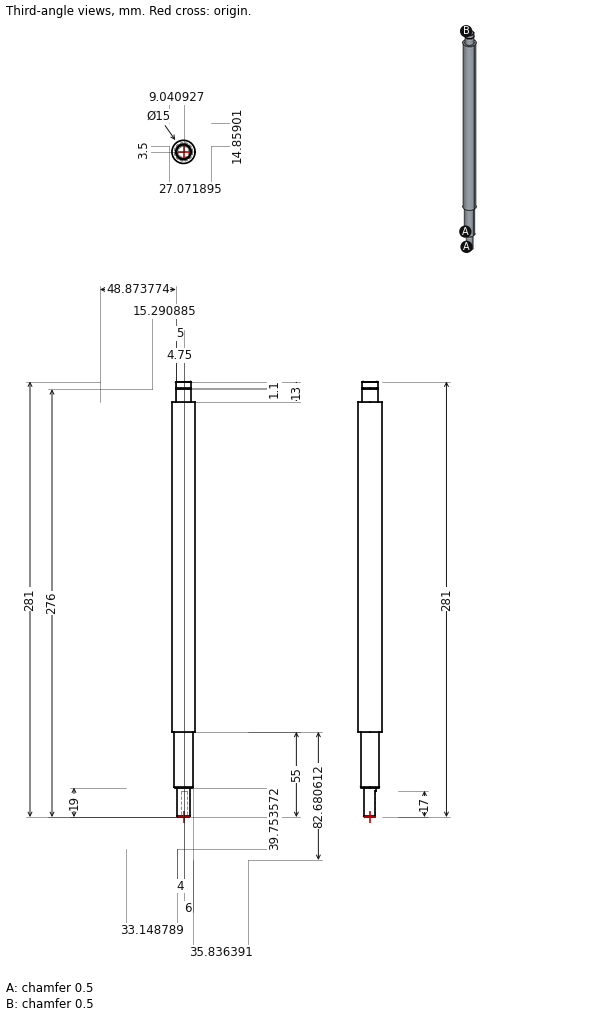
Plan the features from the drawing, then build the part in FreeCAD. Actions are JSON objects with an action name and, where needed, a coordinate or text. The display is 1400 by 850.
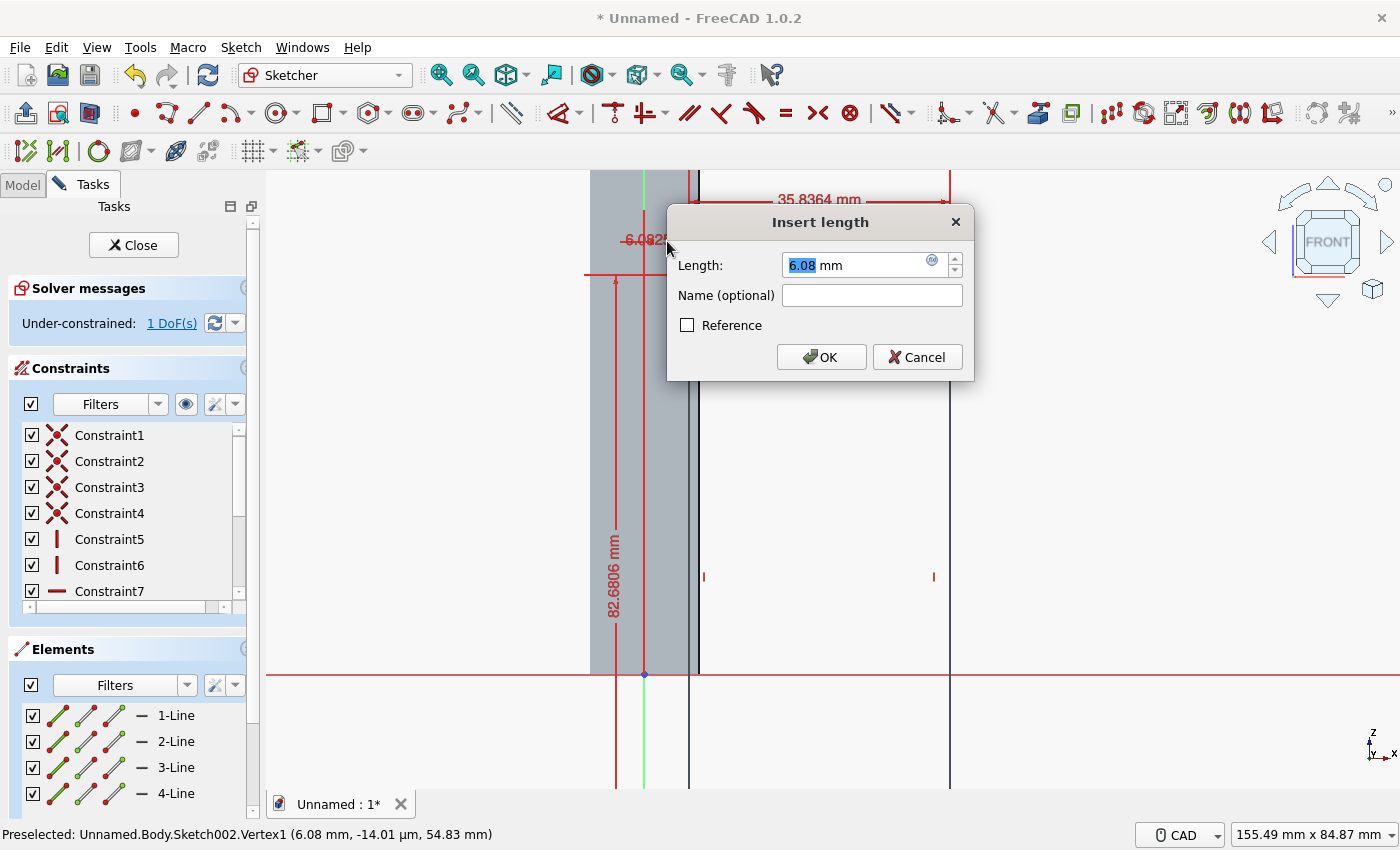
{"action": "type", "text": "6"}
{"action": "key", "text": "Return"}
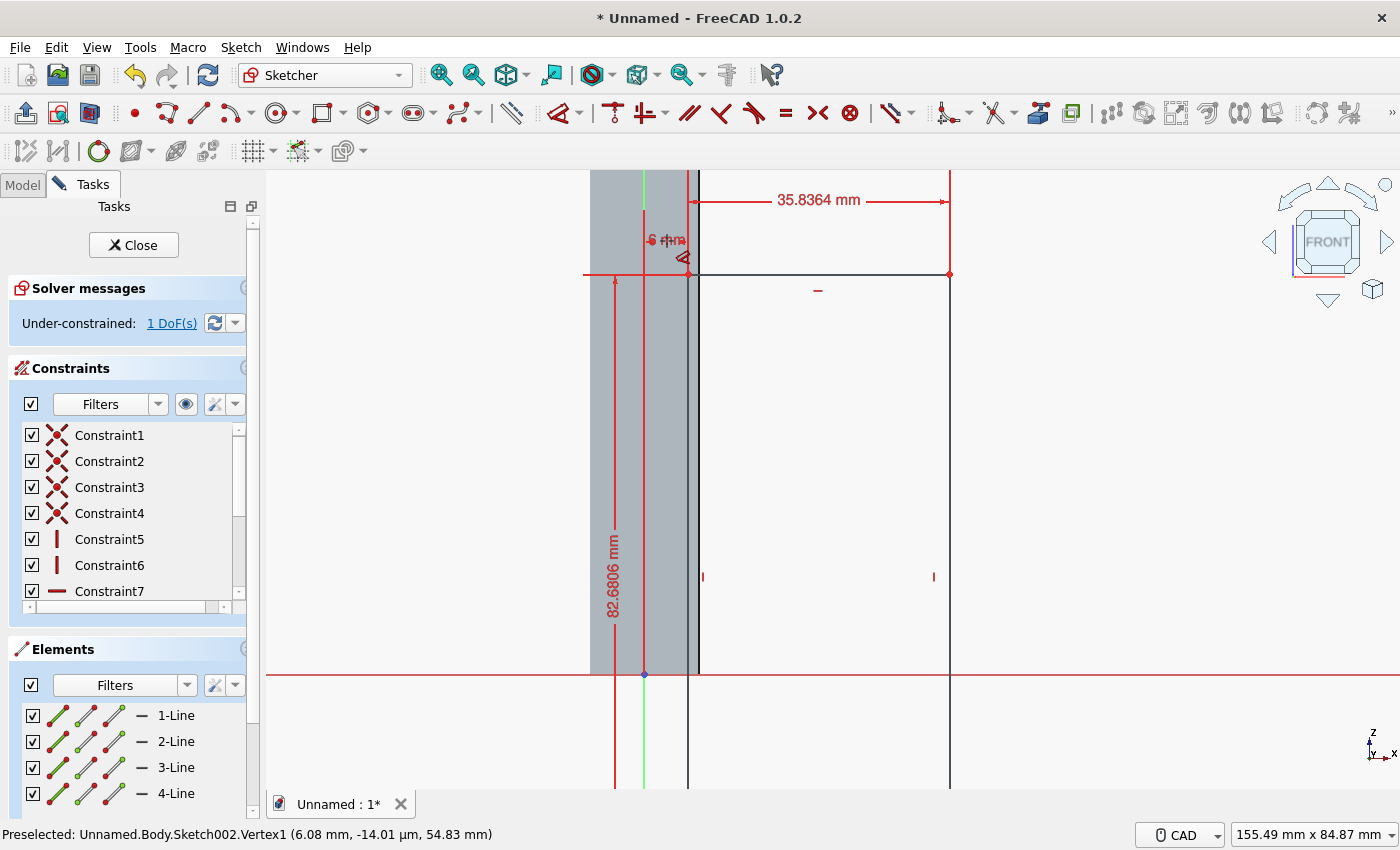
{"action": "left_click", "coordinate": [688, 275]}
{"action": "left_click", "coordinate": [610, 475]}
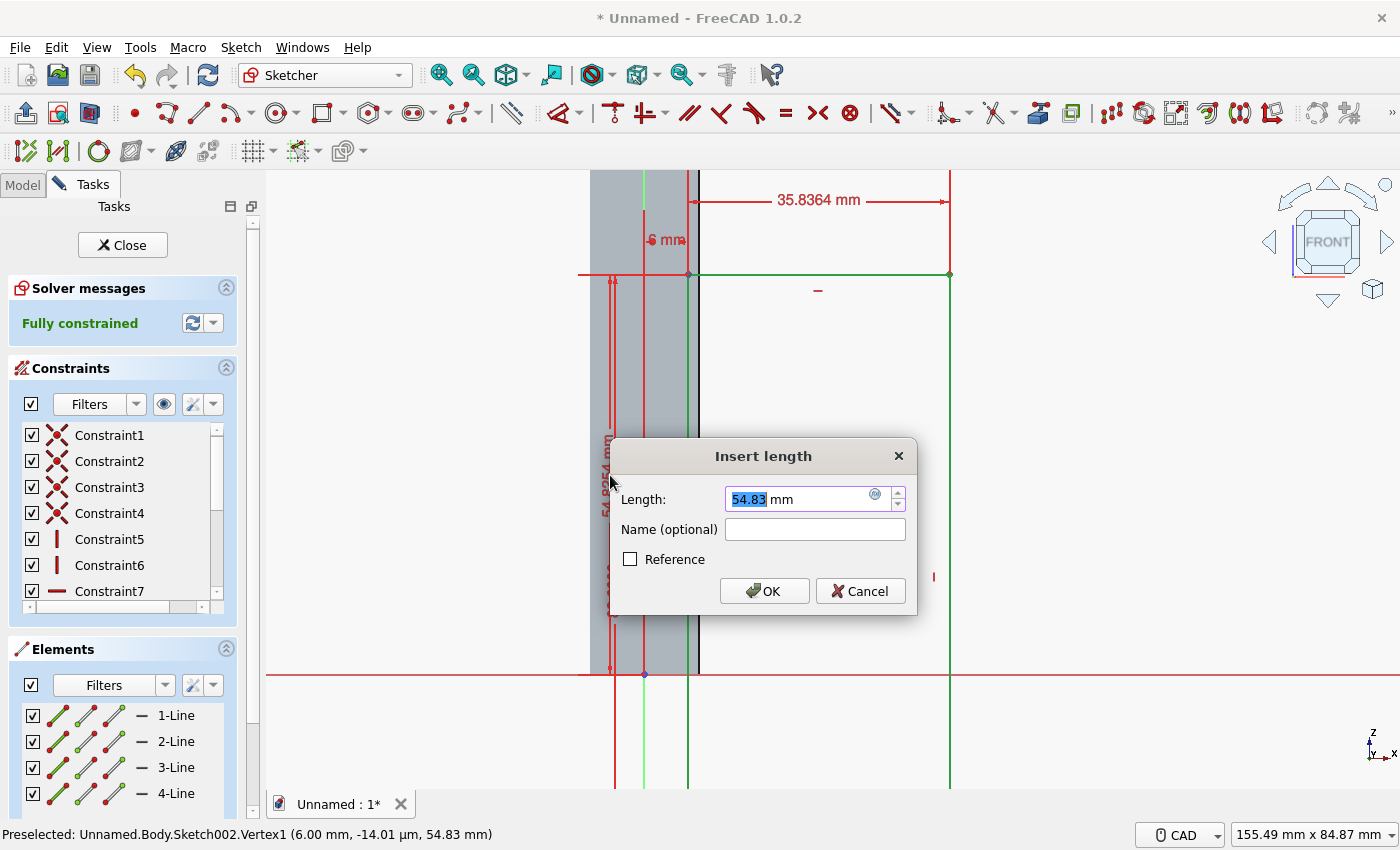
{"action": "type", "text": "55"}
{"action": "key", "text": "Return"}
{"action": "key", "text": "Escape"}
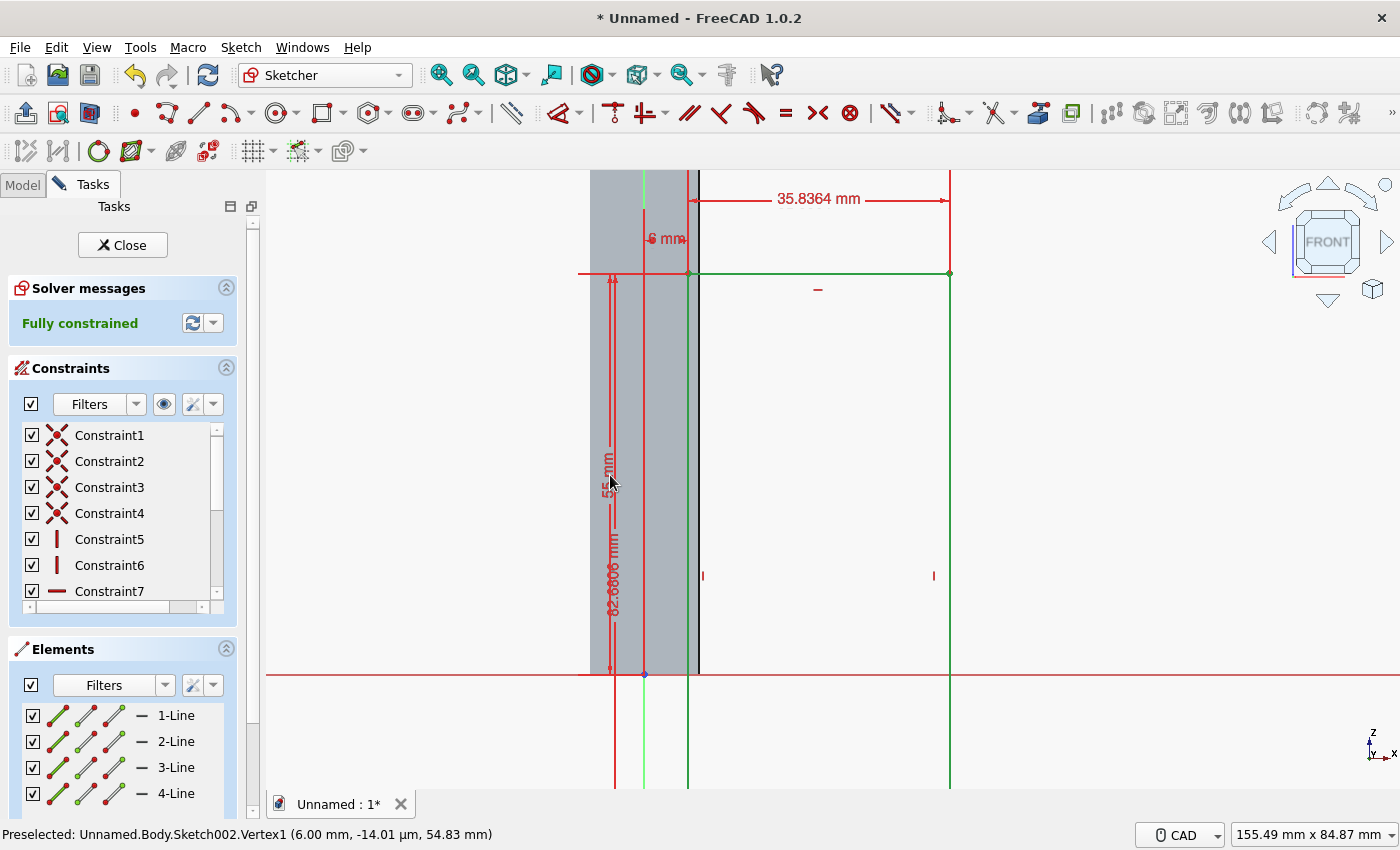
{"action": "left_click", "coordinate": [123, 245]}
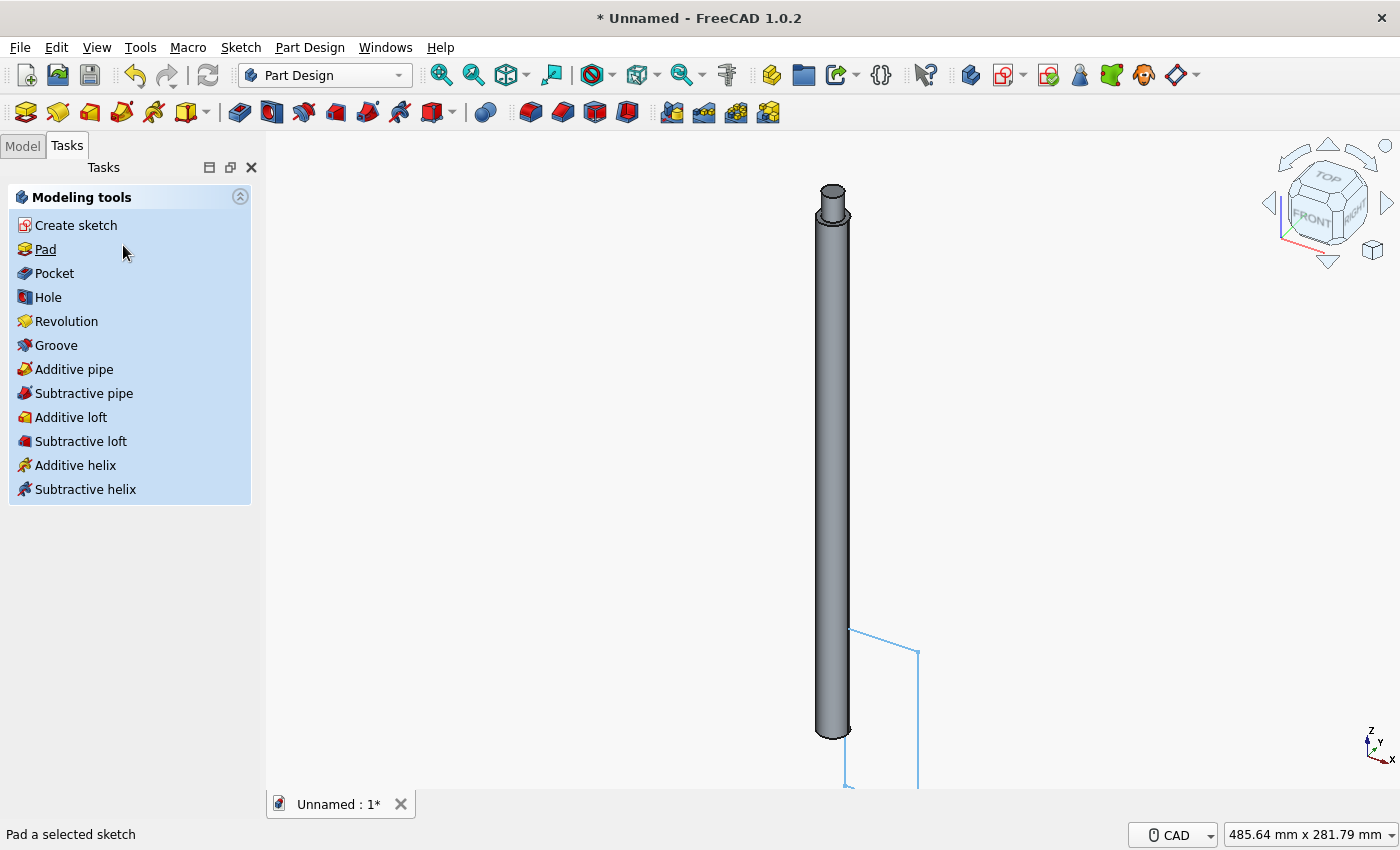
{"action": "left_click", "coordinate": [304, 112]}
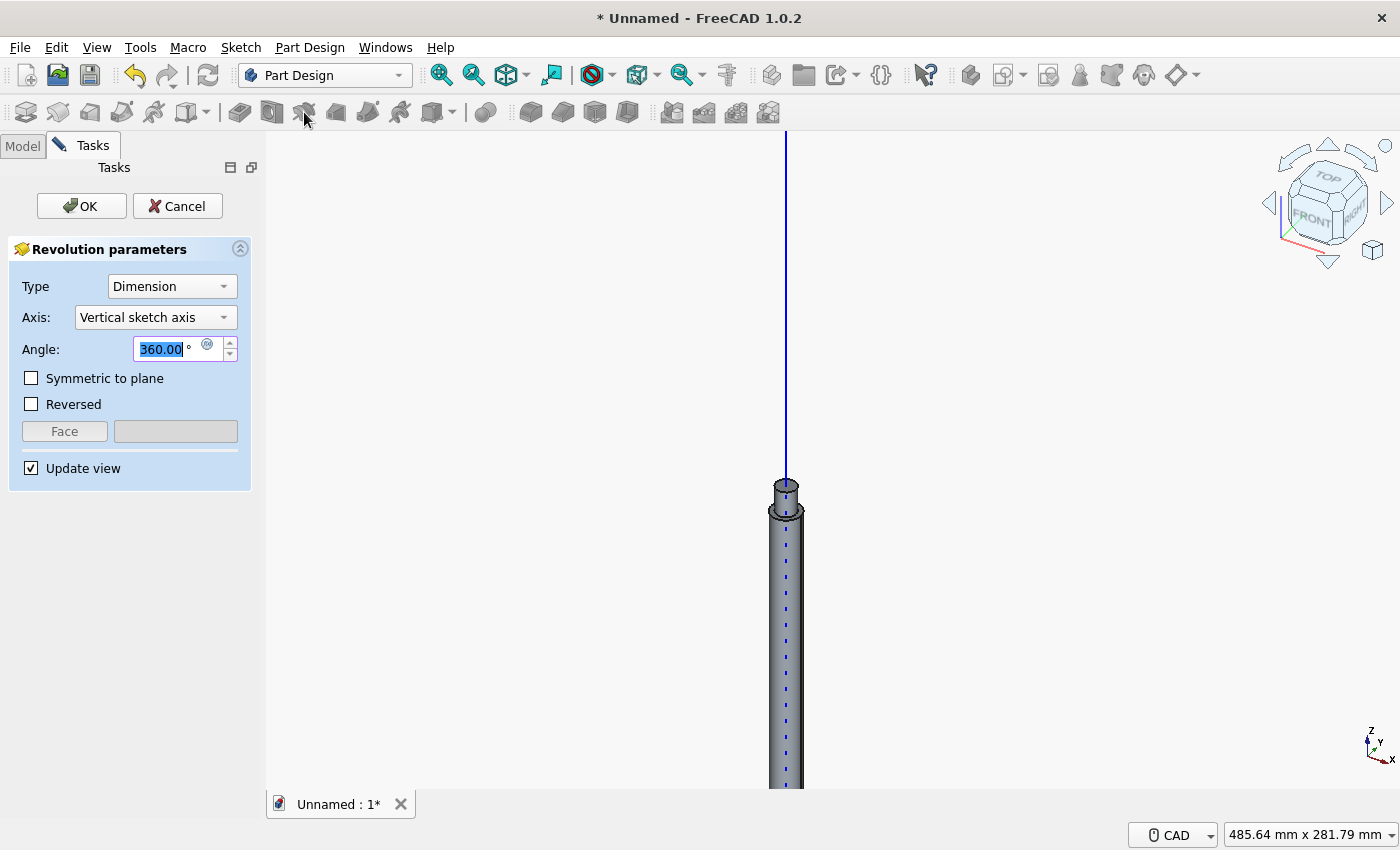
{"action": "left_click", "coordinate": [82, 206]}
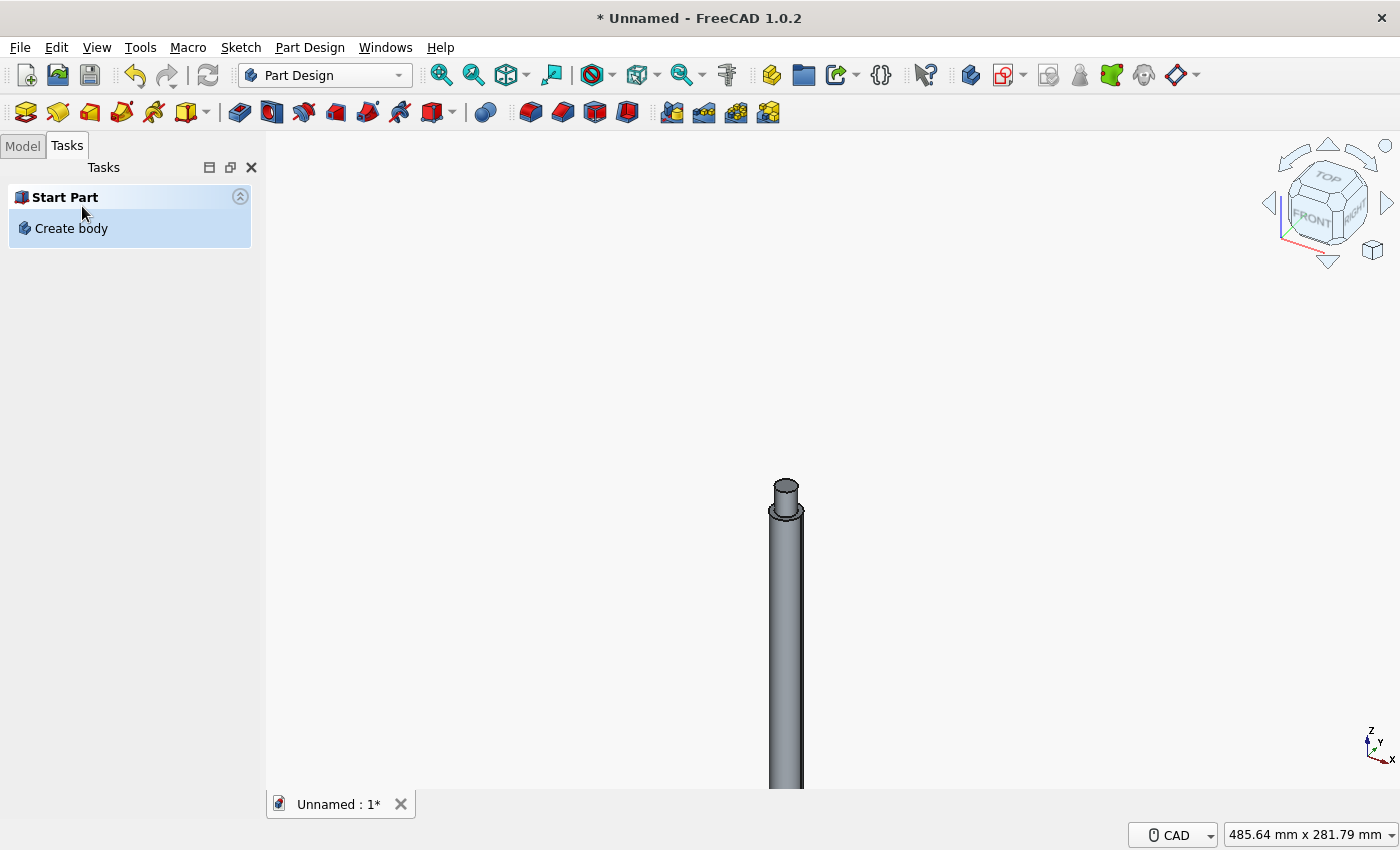
{"action": "left_click", "coordinate": [442, 76]}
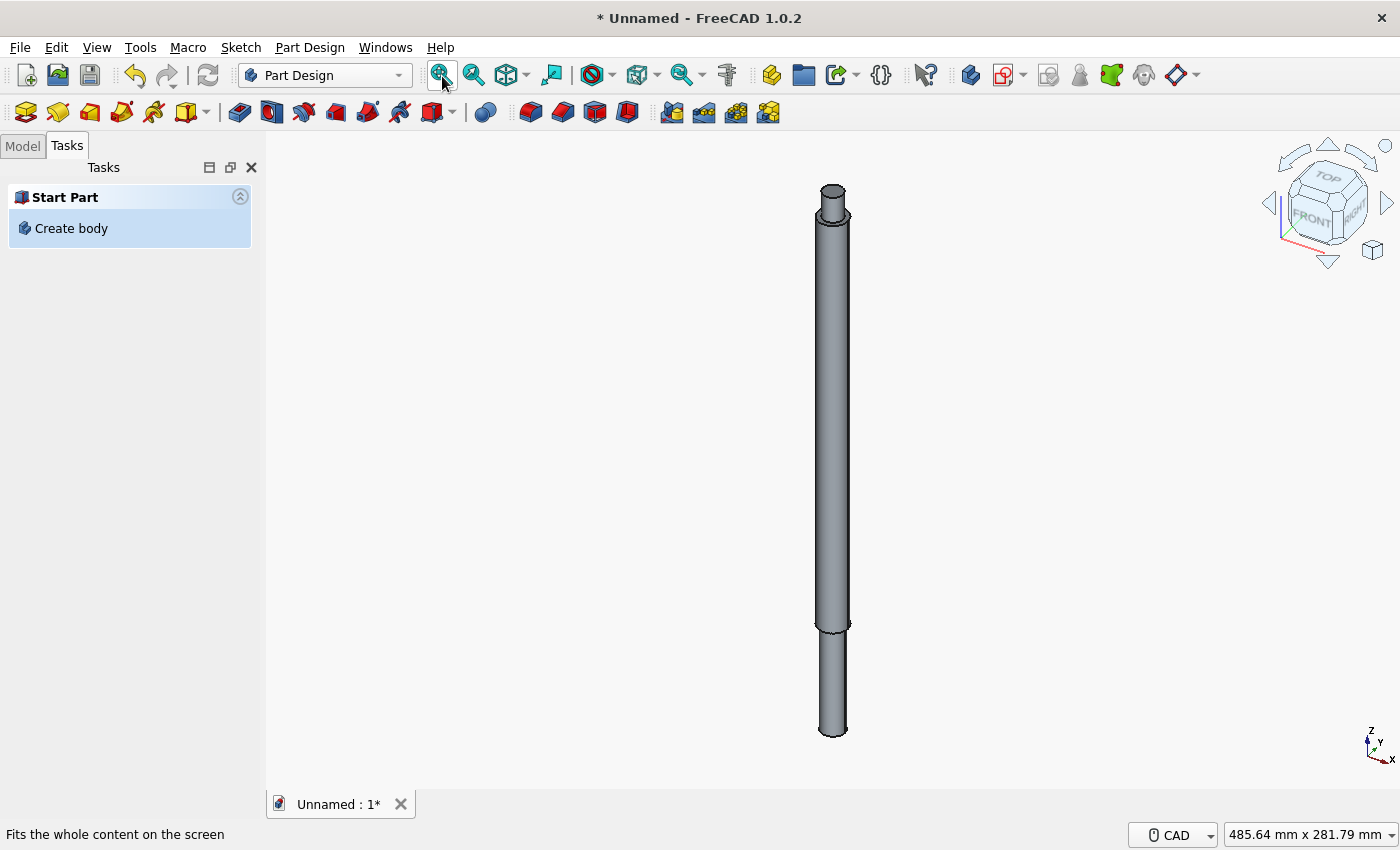
{"action": "left_click", "coordinate": [1004, 76]}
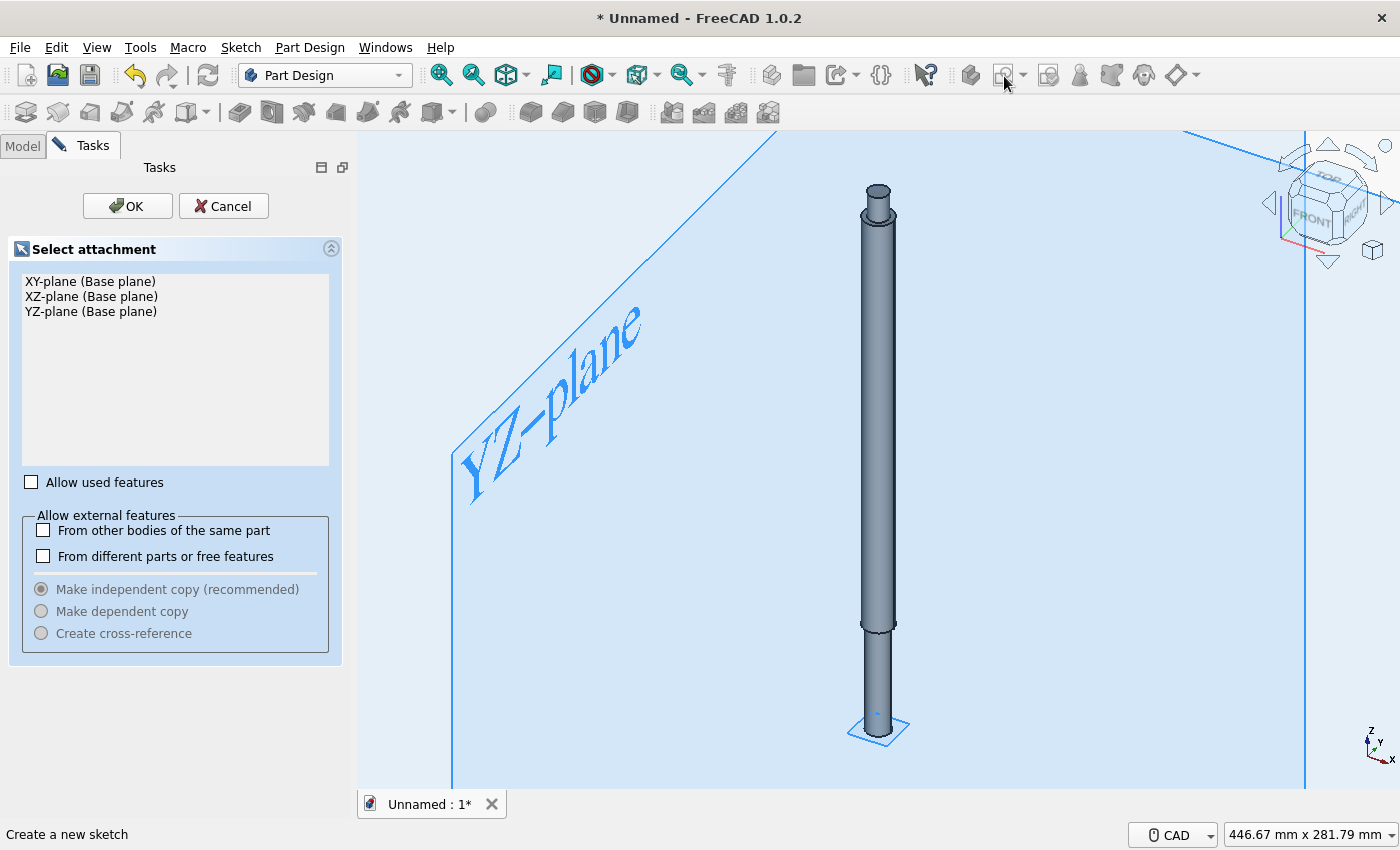
{"action": "left_click", "coordinate": [82, 296]}